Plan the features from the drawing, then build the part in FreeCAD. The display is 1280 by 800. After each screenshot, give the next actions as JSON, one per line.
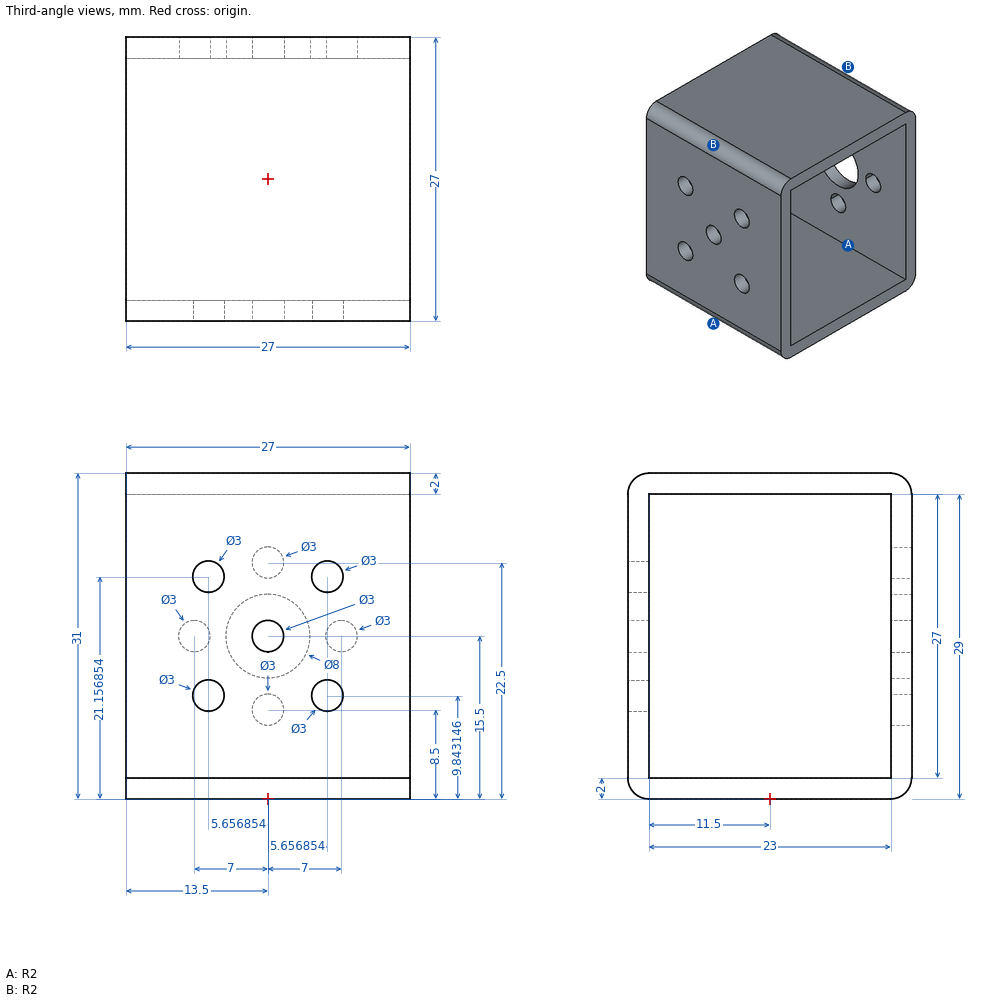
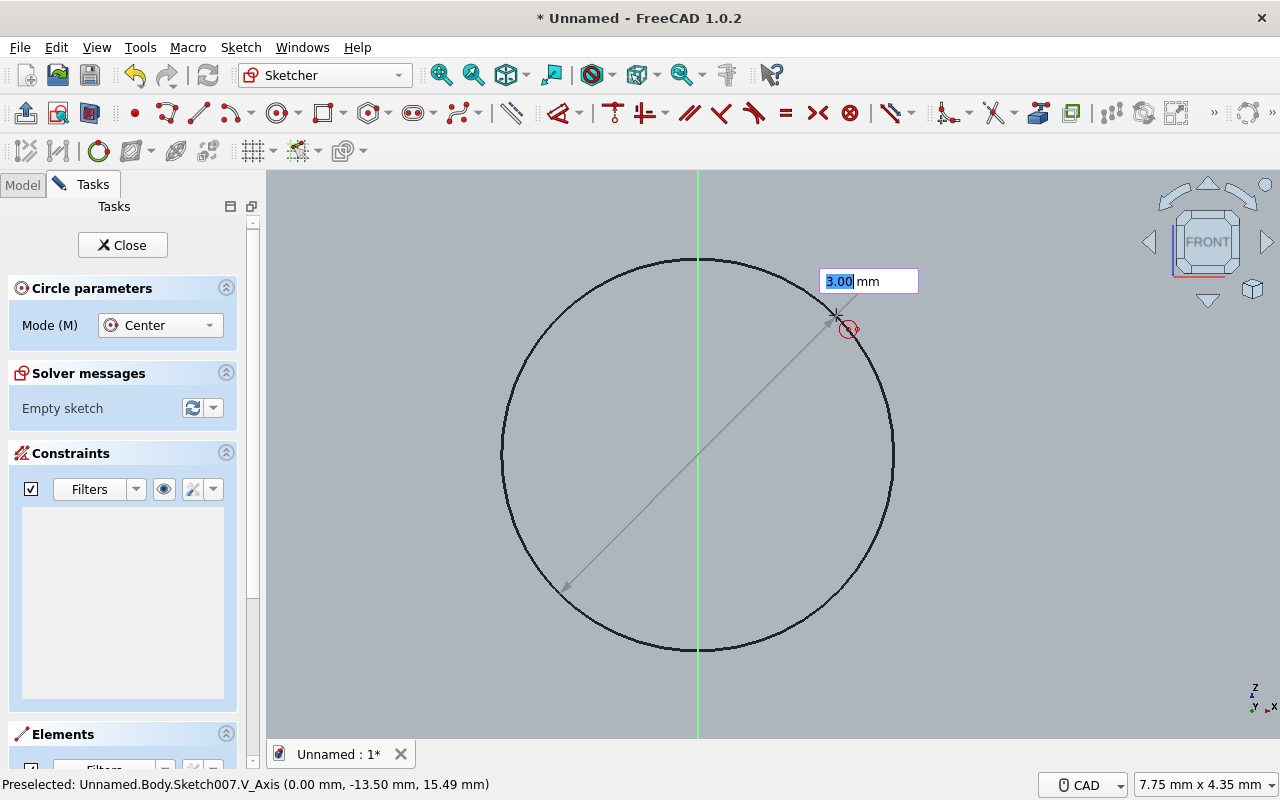
{"action": "type", "text": "3"}
{"action": "key", "text": "Return"}
{"action": "key", "text": "Escape"}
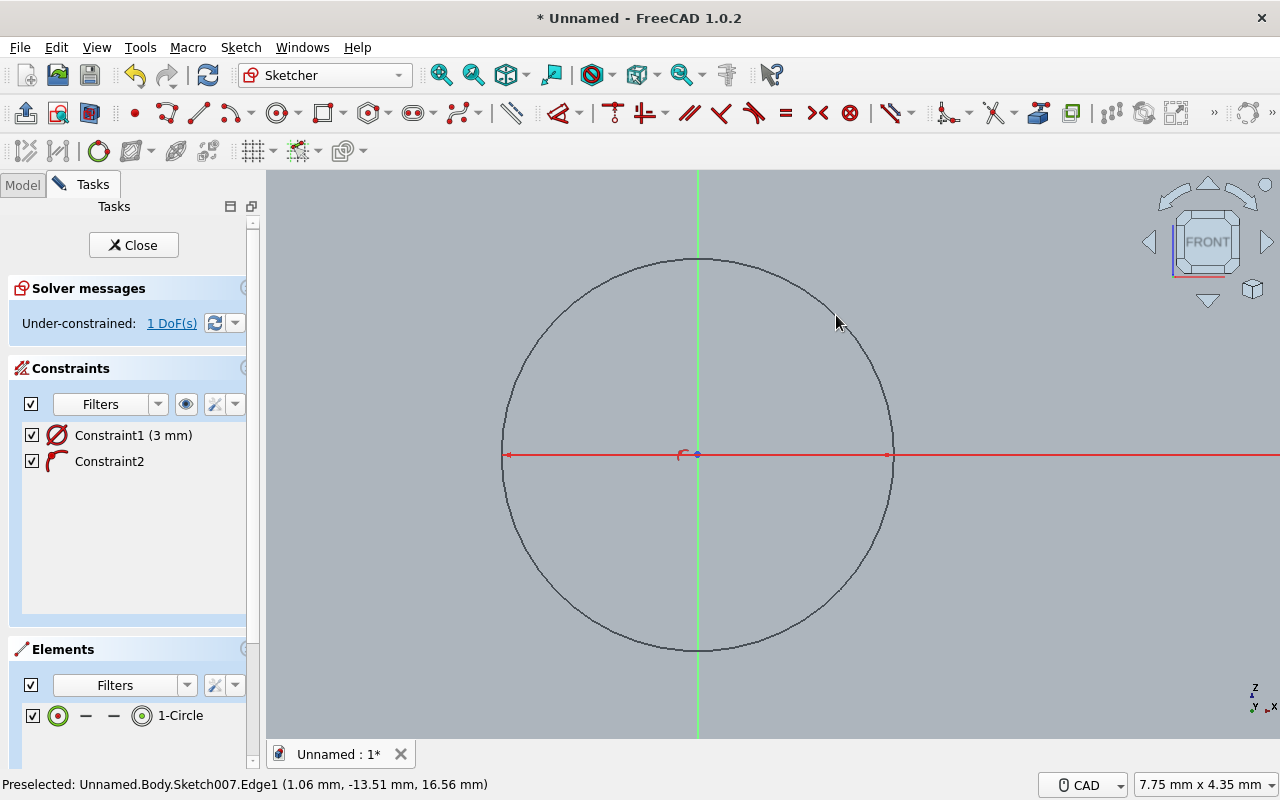
{"action": "left_click", "coordinate": [558, 114]}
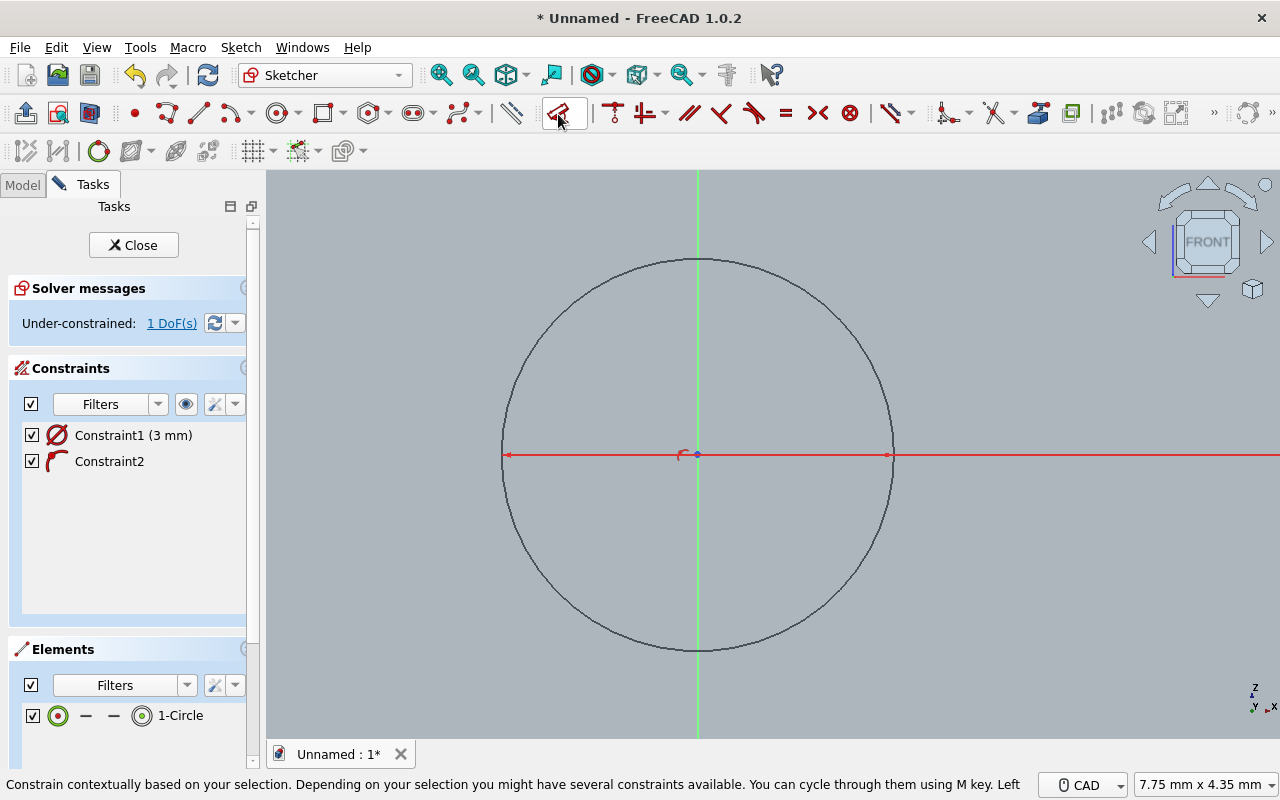
{"action": "left_click", "coordinate": [698, 455]}
{"action": "left_click", "coordinate": [732, 583]}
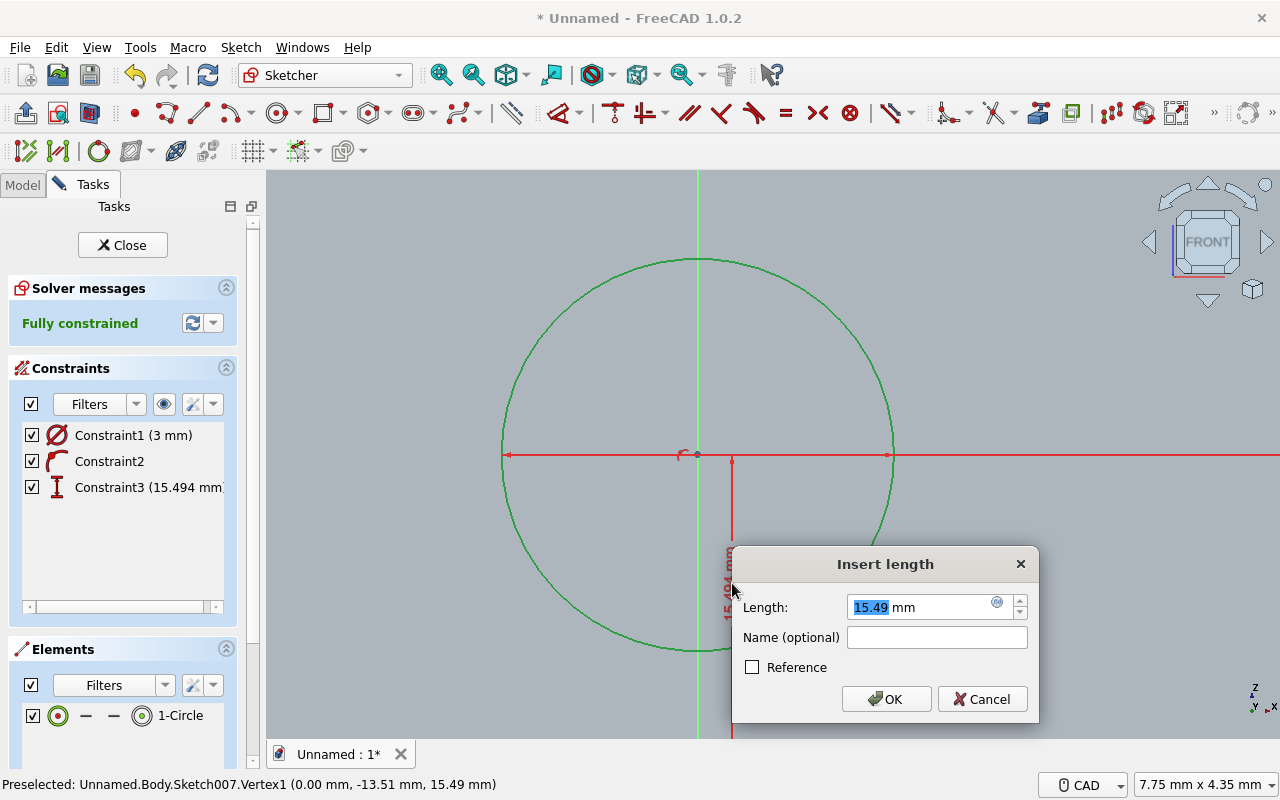
{"action": "type", "text": "15.5"}
{"action": "key", "text": "Return"}
{"action": "key", "text": "Escape"}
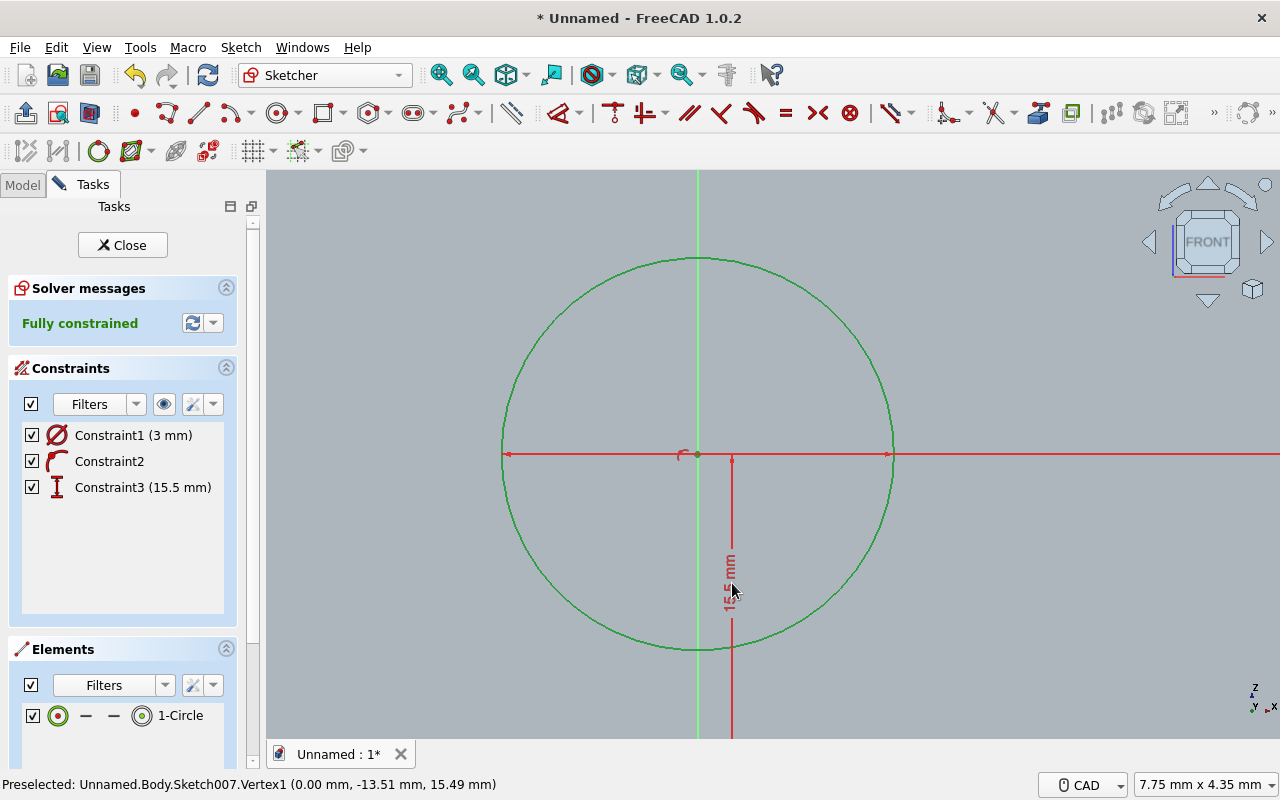
{"action": "left_click", "coordinate": [123, 245]}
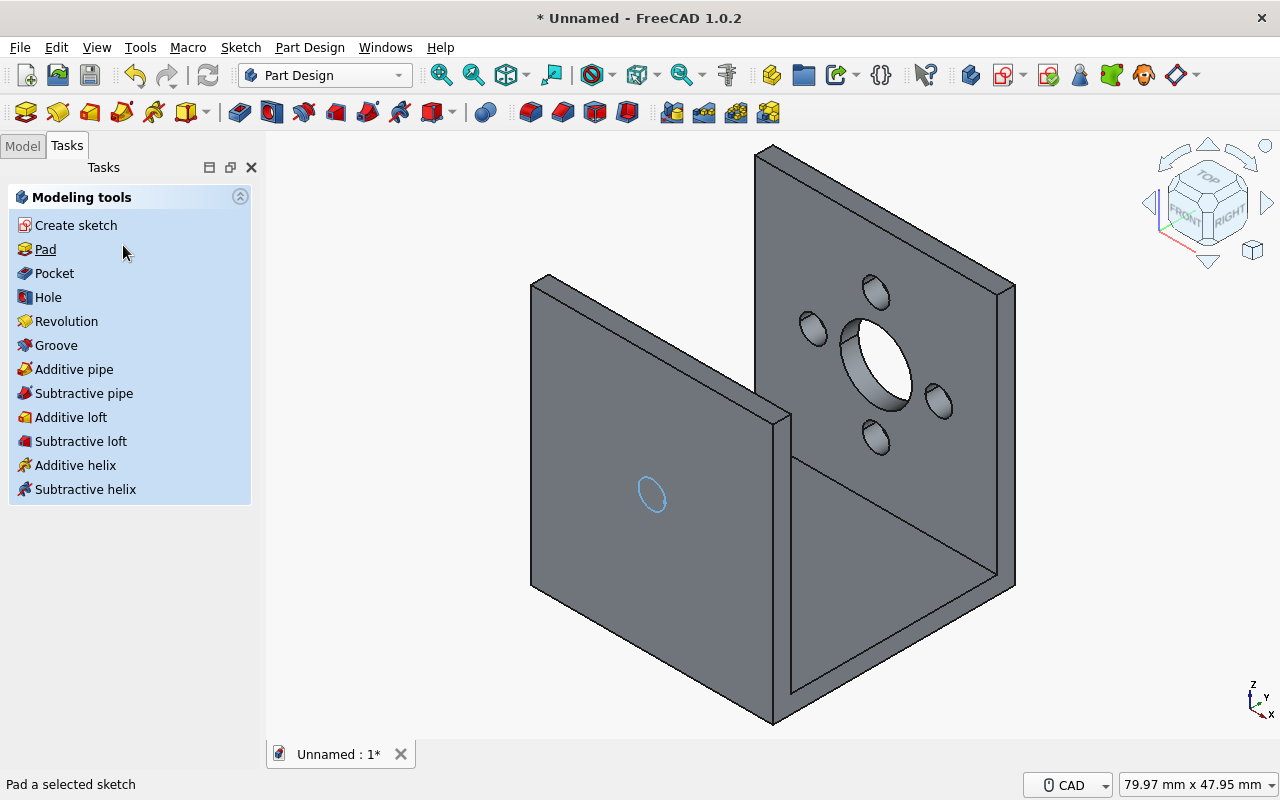
{"action": "left_click", "coordinate": [240, 112]}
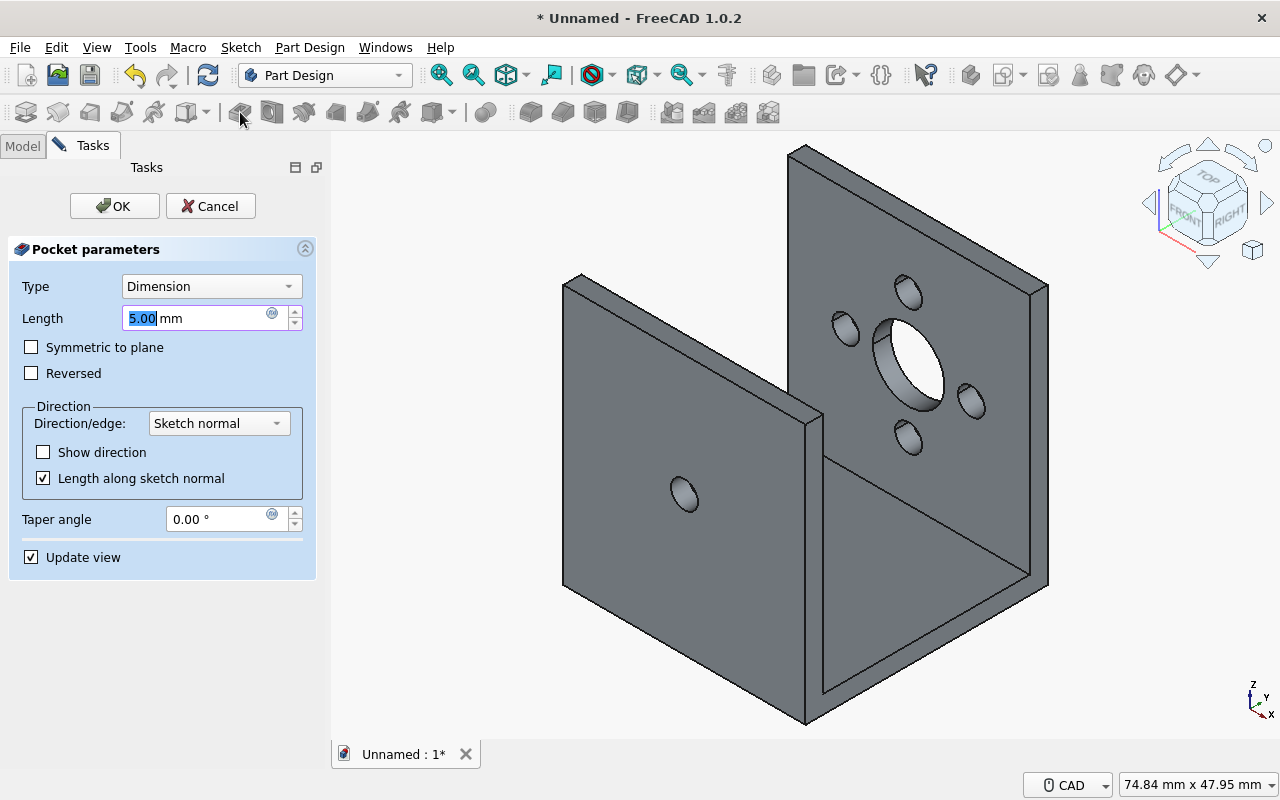
{"action": "left_click", "coordinate": [212, 286]}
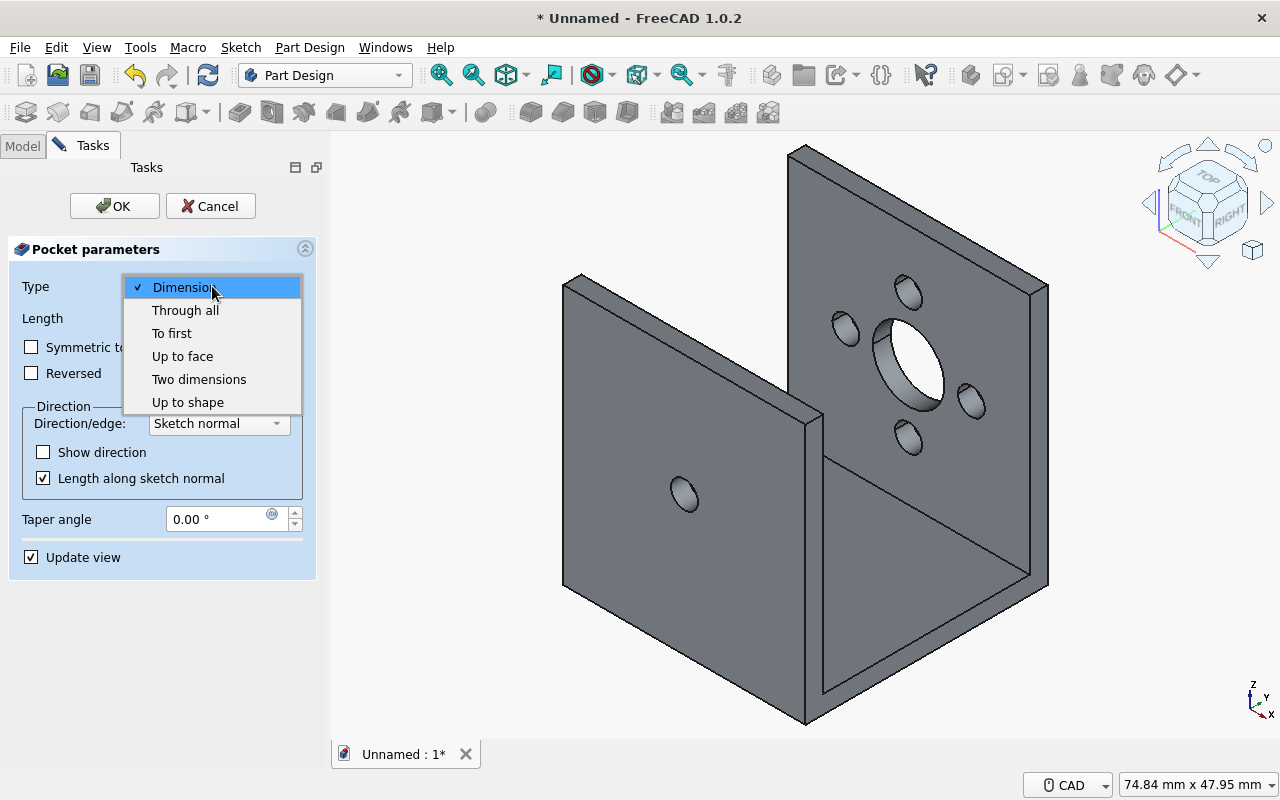
{"action": "left_click", "coordinate": [212, 334]}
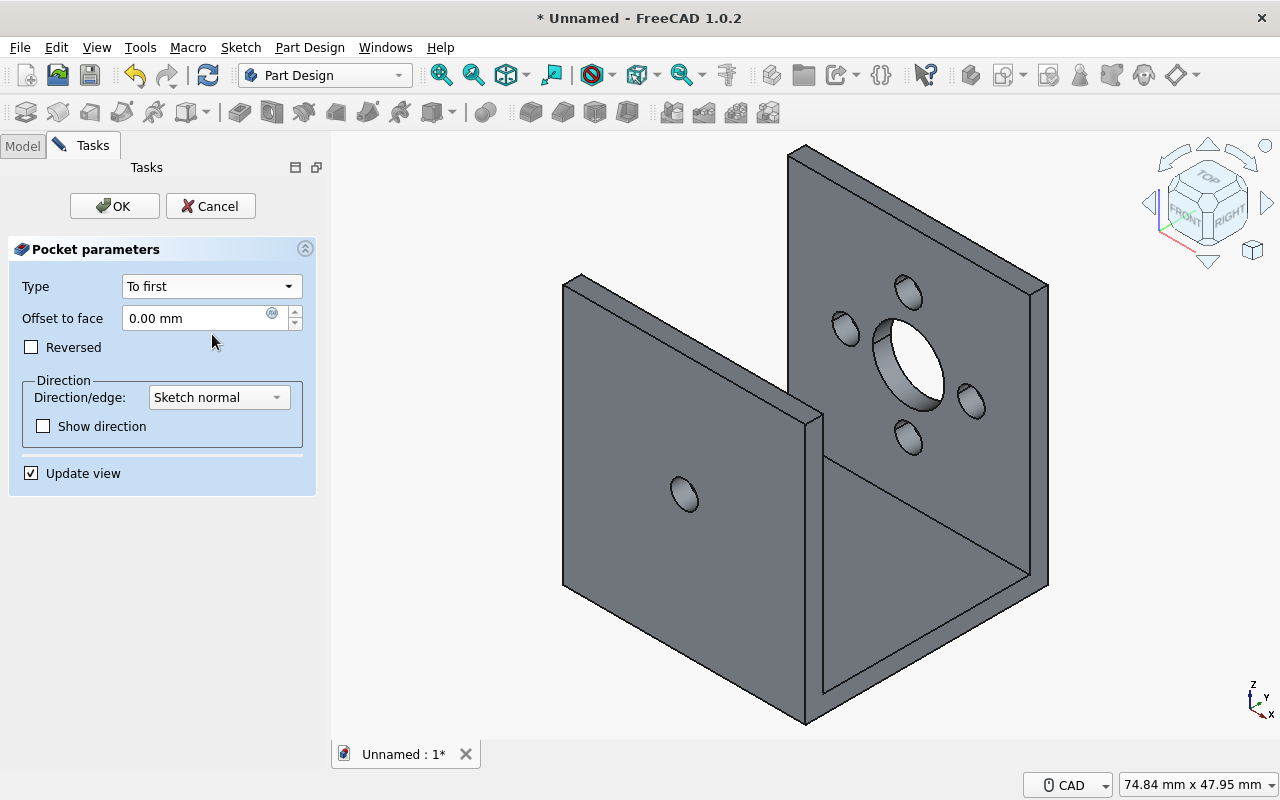
{"action": "left_click", "coordinate": [115, 206]}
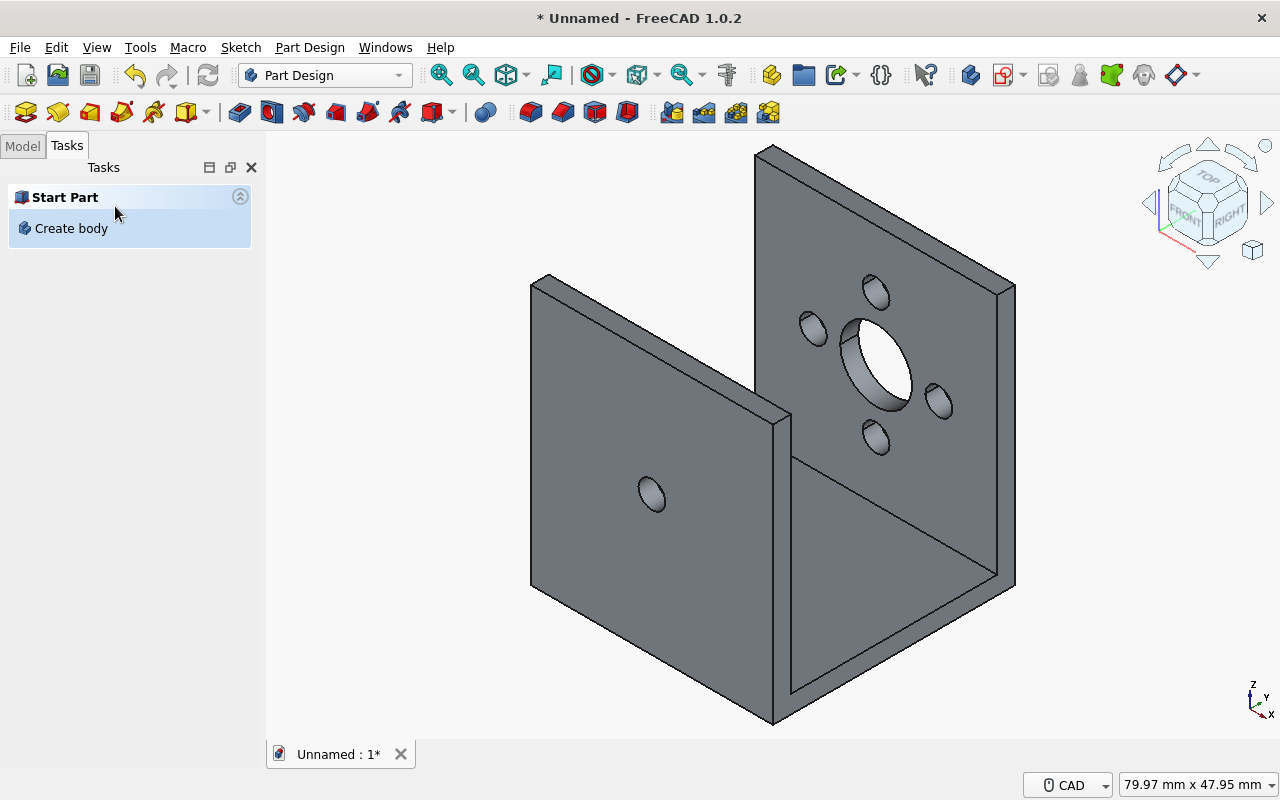
{"action": "left_click", "coordinate": [687, 438]}